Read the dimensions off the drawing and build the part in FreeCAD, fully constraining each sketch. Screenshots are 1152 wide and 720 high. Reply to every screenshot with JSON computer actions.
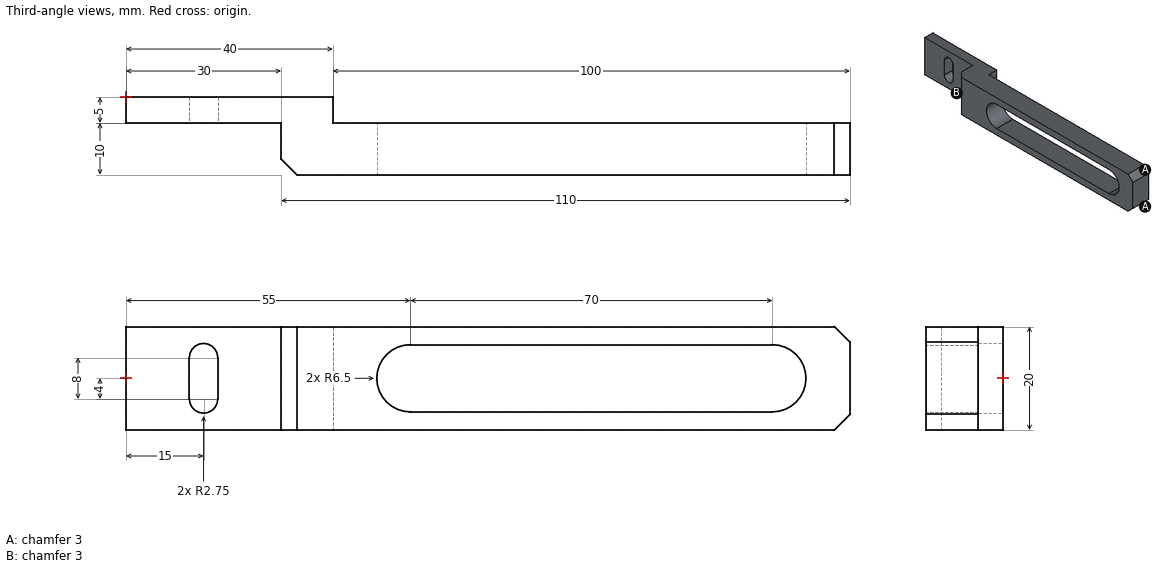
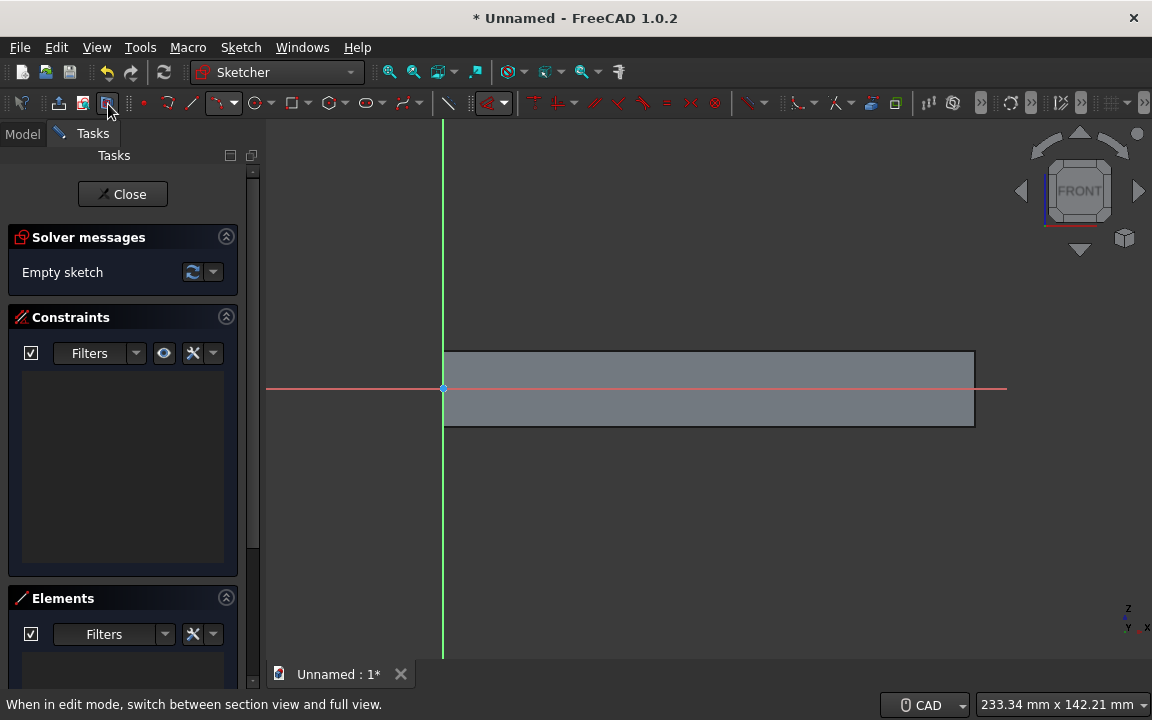
{"action": "left_click", "coordinate": [366, 104]}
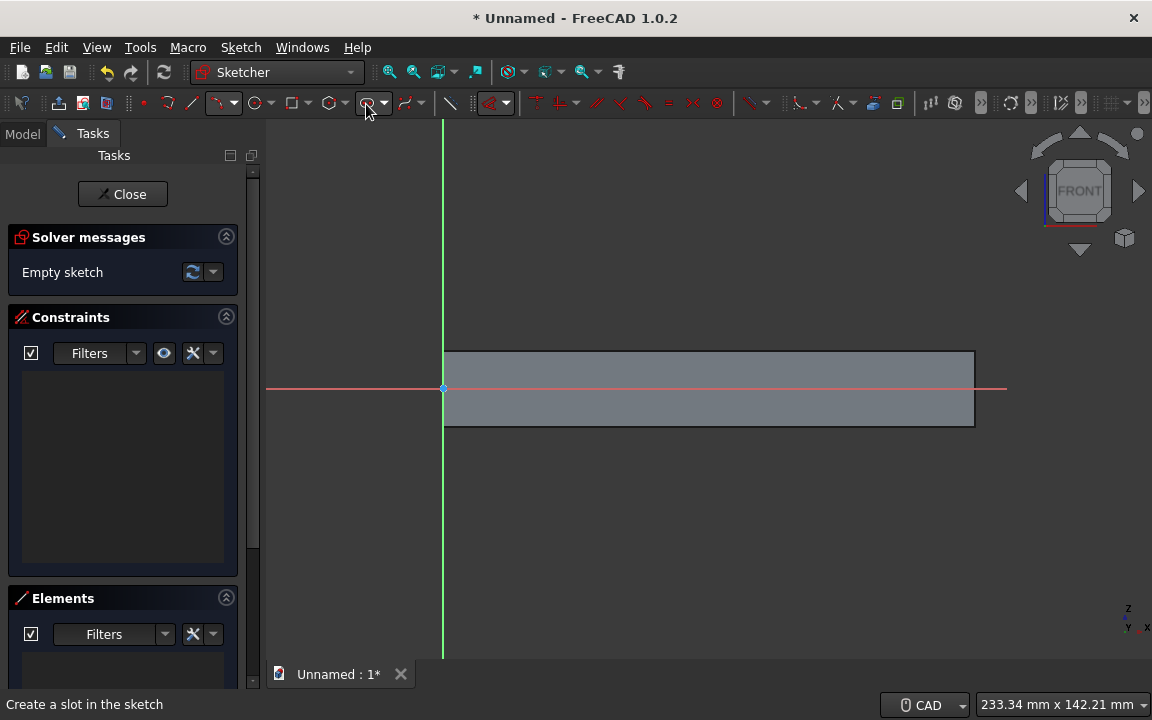
{"action": "left_click", "coordinate": [652, 389]}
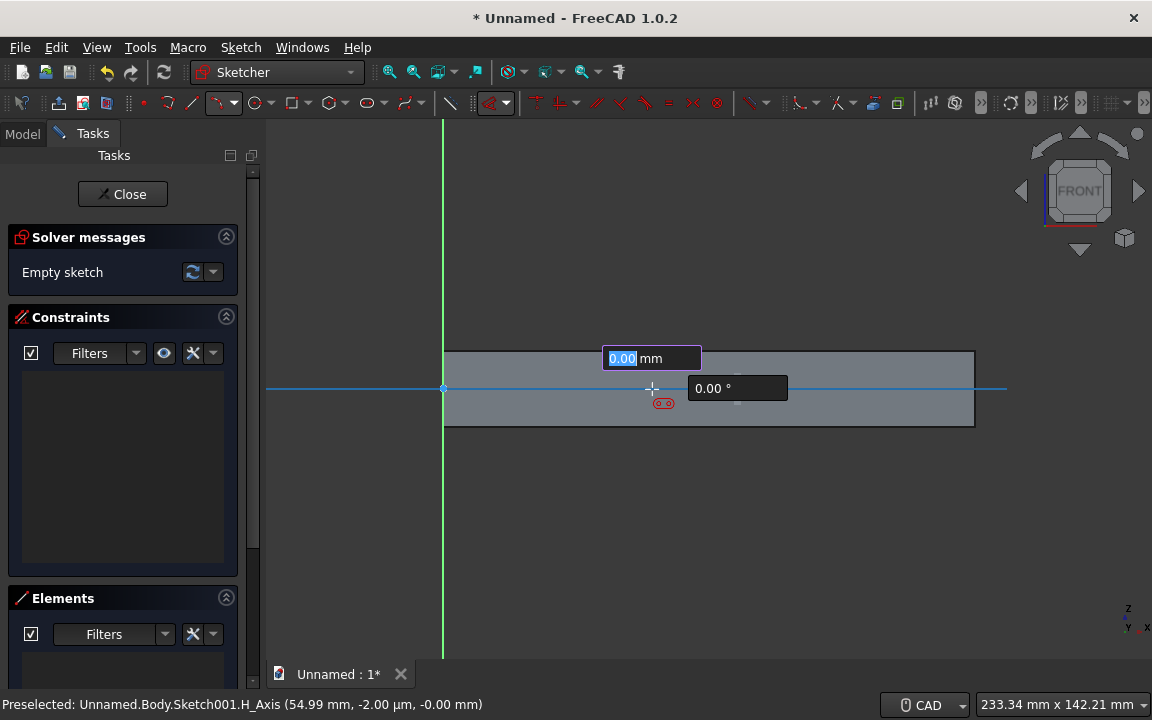
{"action": "left_click", "coordinate": [918, 380]}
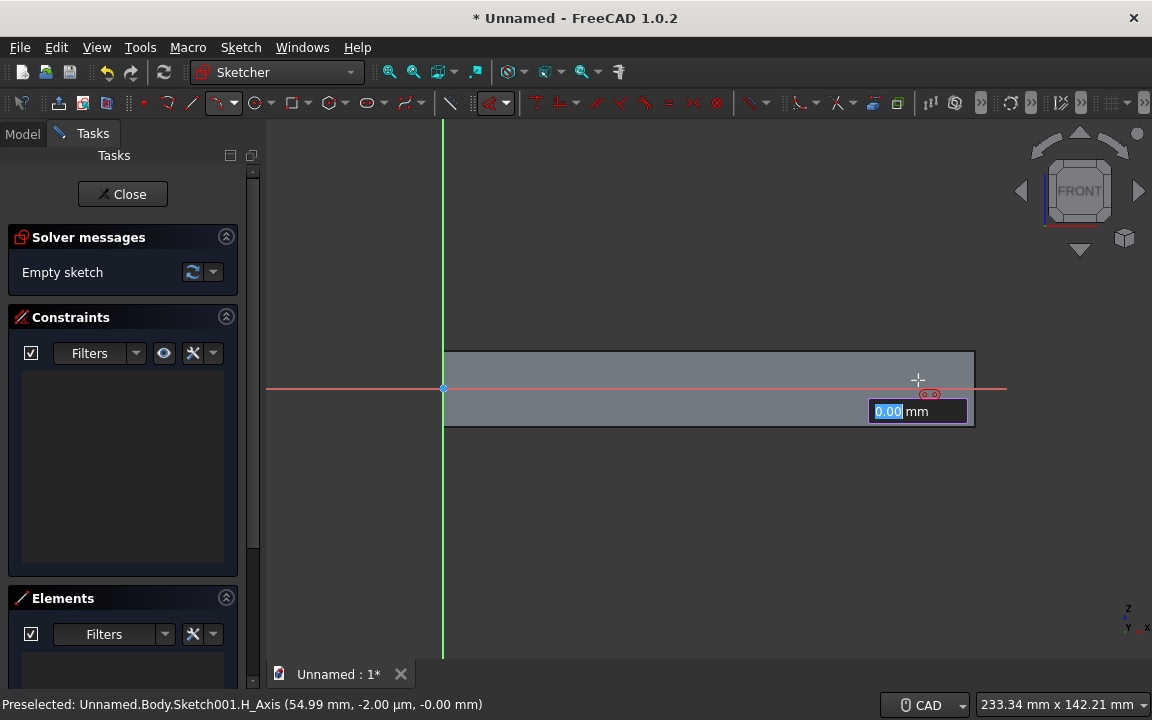
{"action": "left_click", "coordinate": [785, 414]}
{"action": "key", "text": "Escape"}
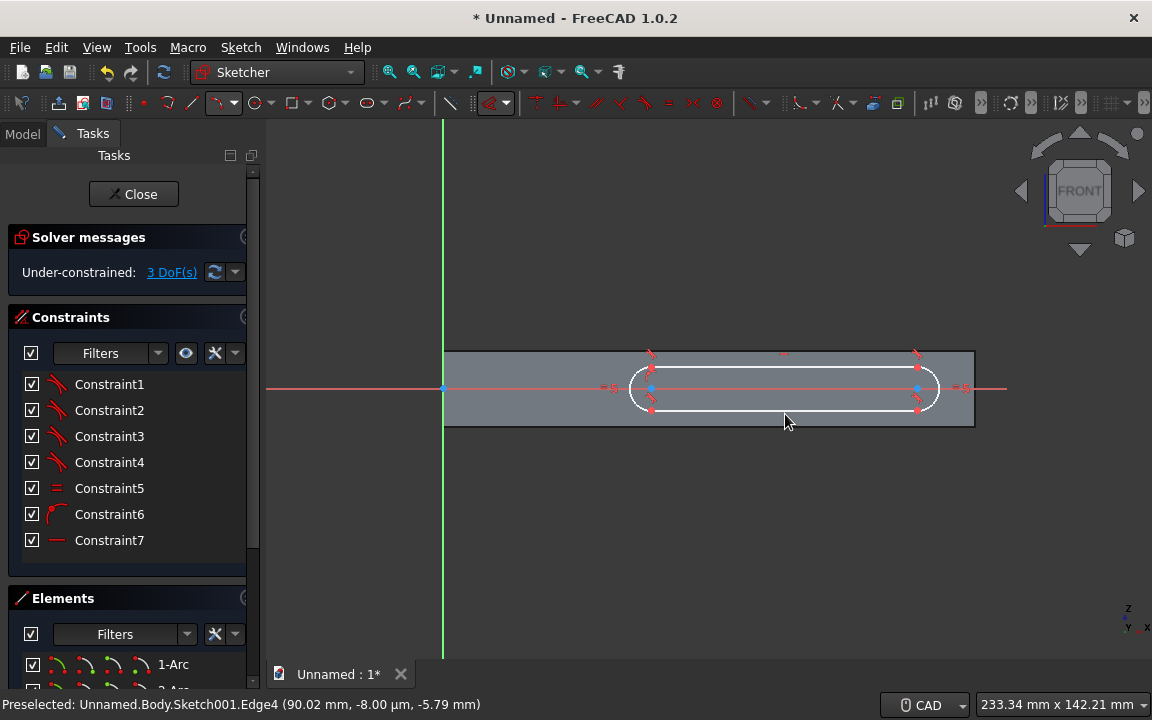
{"action": "scroll", "coordinate": [634, 376], "scroll_direction": "up", "scroll_amount": 3}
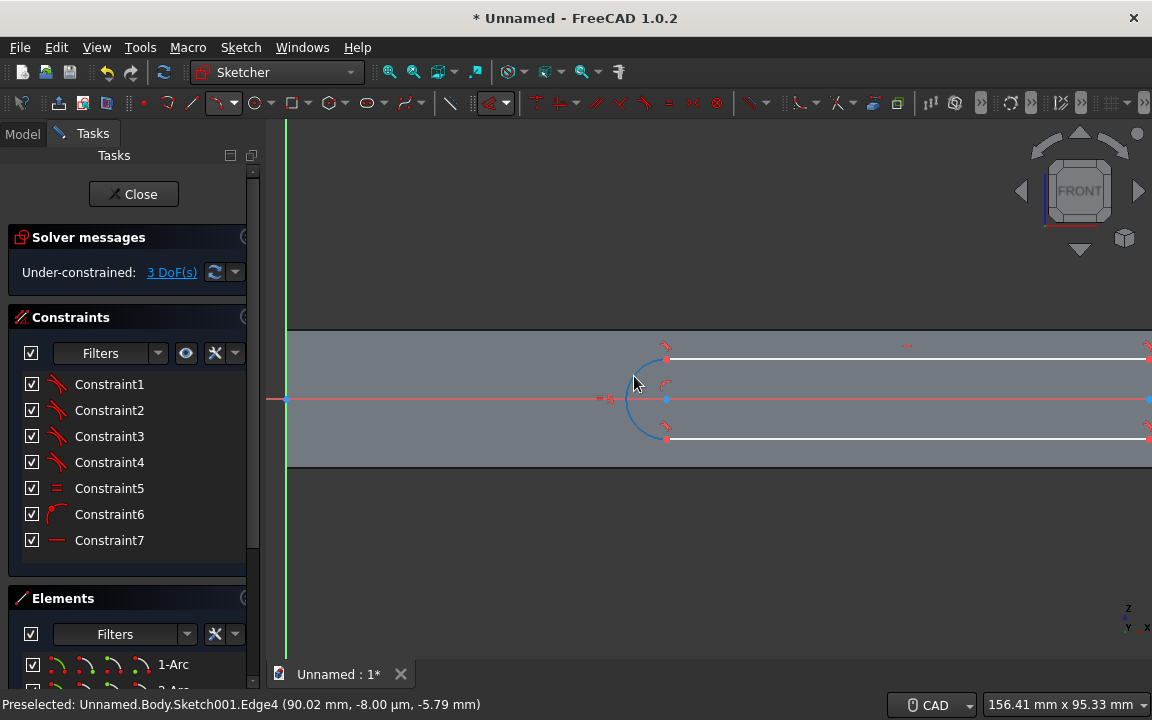
{"action": "left_click", "coordinate": [634, 376]}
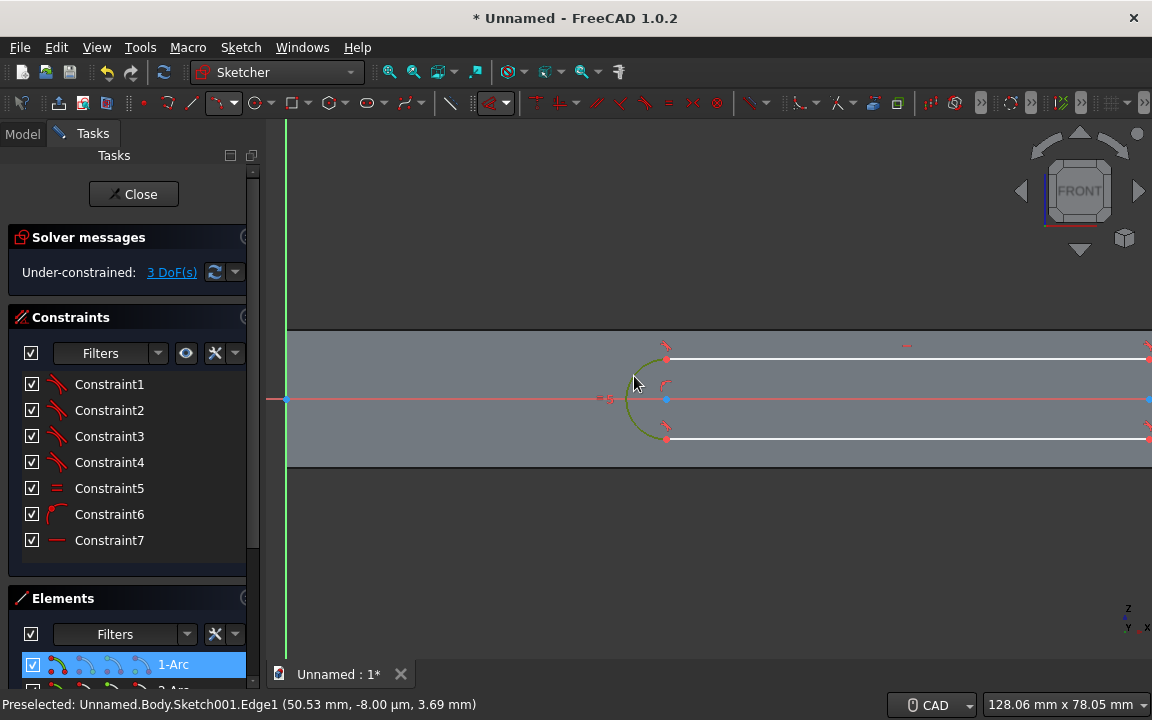
{"action": "left_click", "coordinate": [508, 104]}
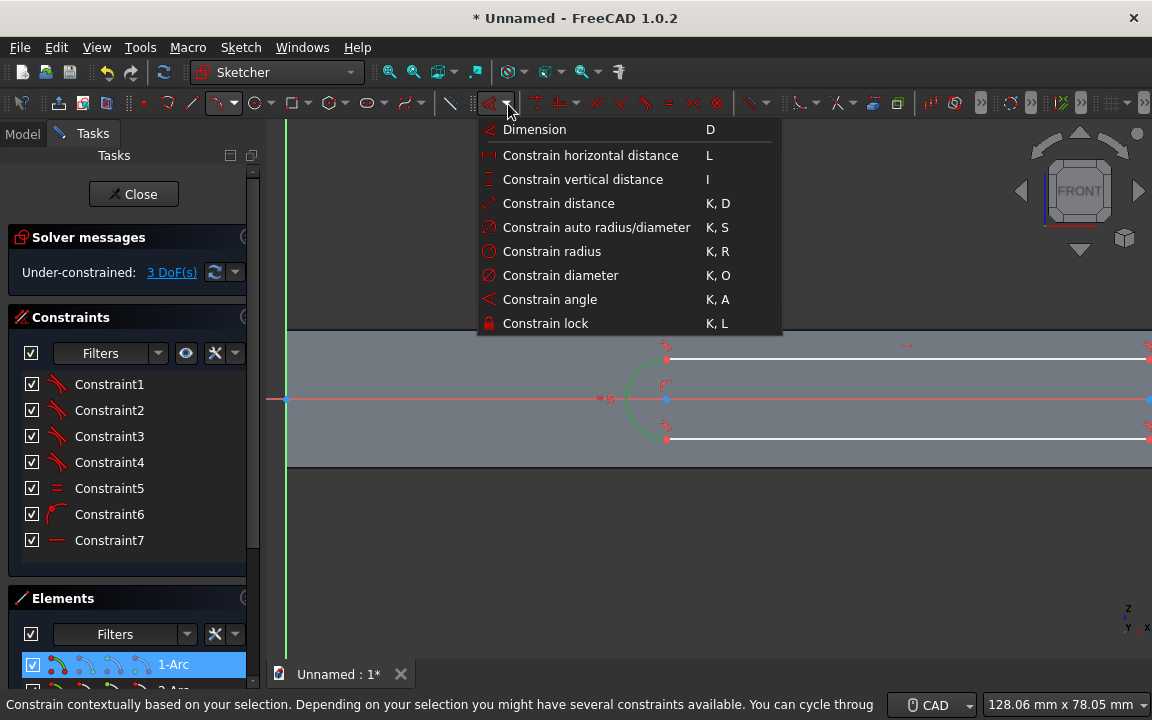
{"action": "left_click", "coordinate": [630, 251]}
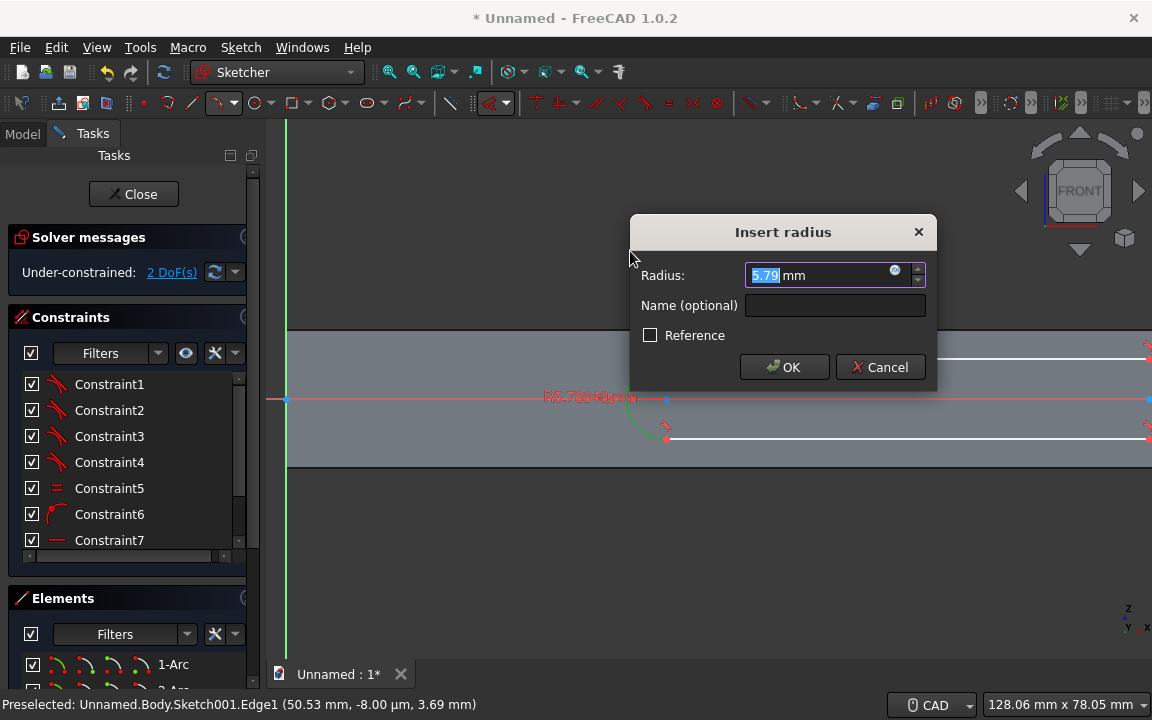
{"action": "type", "text": "6.5"}
{"action": "key", "text": "Return"}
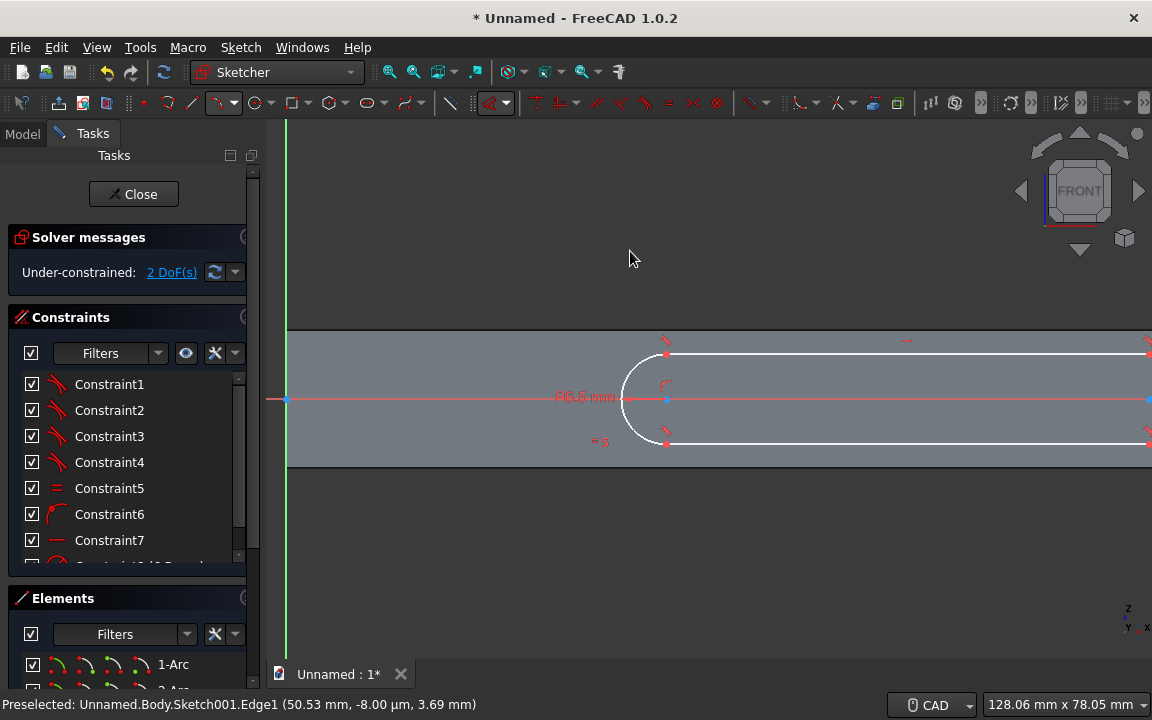
{"action": "left_click", "coordinate": [811, 354]}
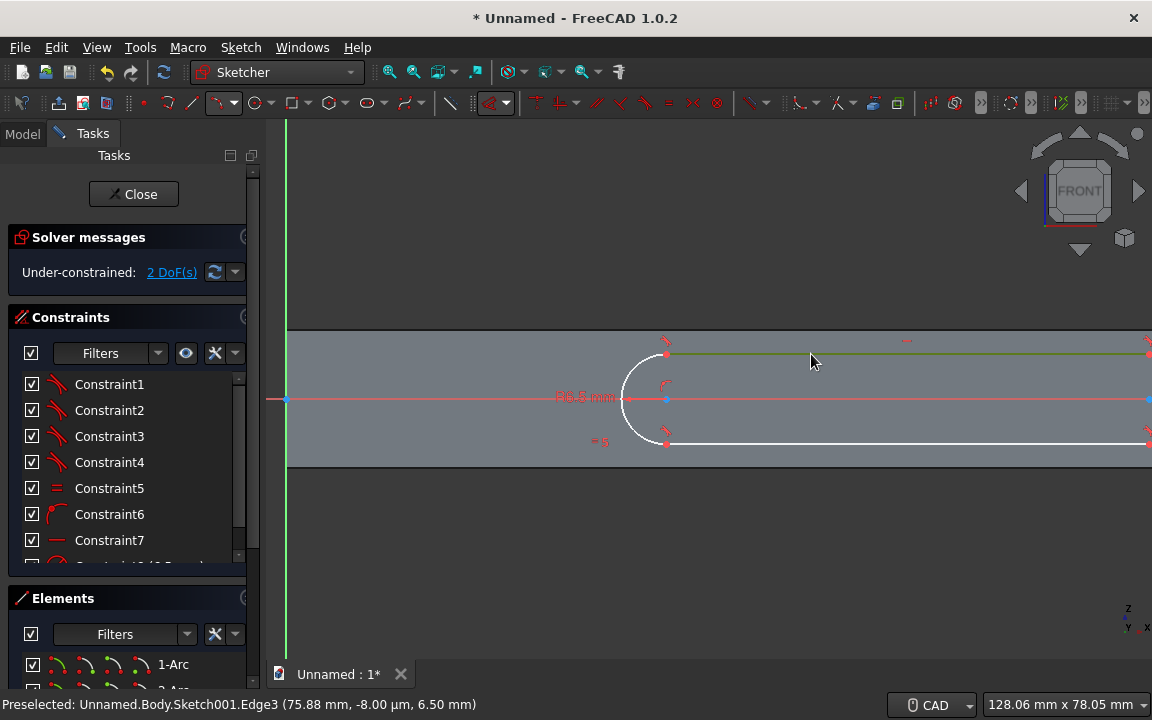
{"action": "key", "text": "l"}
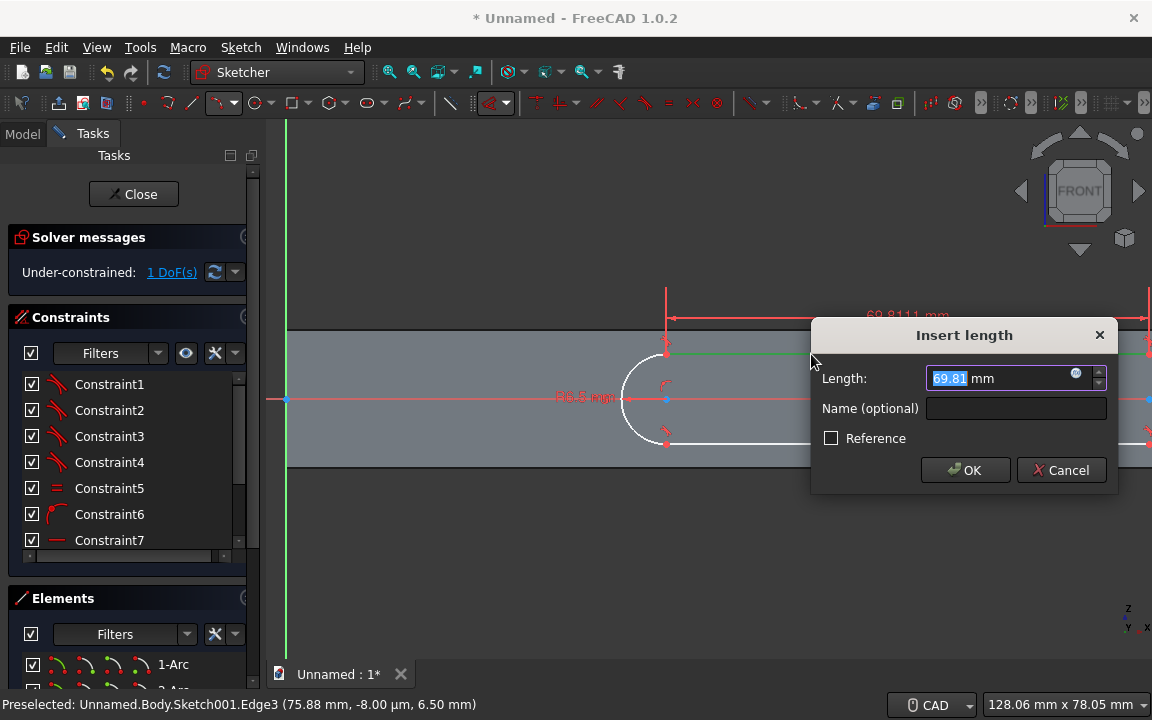
{"action": "type", "text": "70"}
{"action": "key", "text": "Return"}